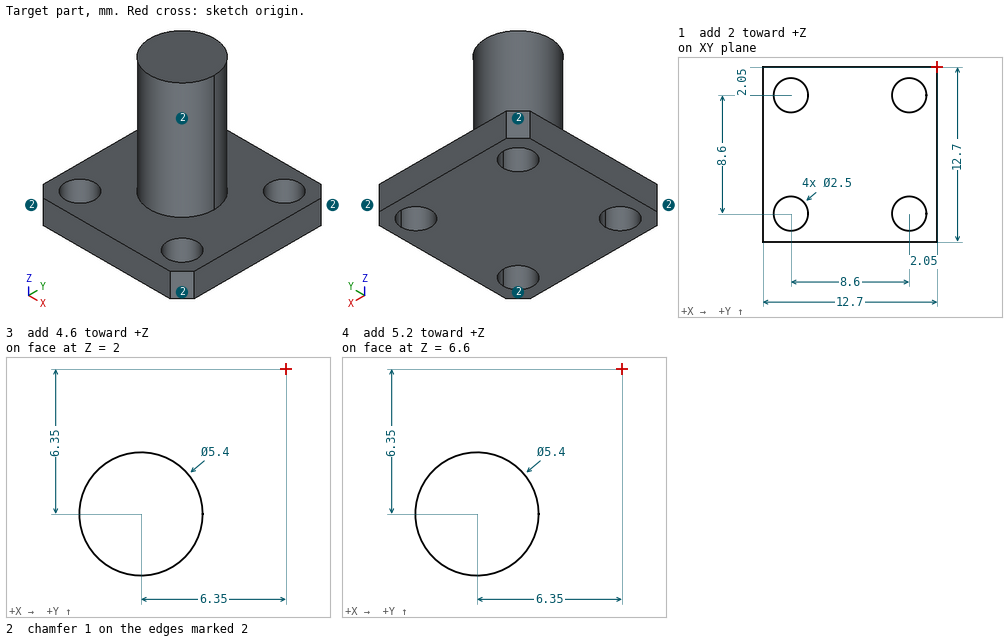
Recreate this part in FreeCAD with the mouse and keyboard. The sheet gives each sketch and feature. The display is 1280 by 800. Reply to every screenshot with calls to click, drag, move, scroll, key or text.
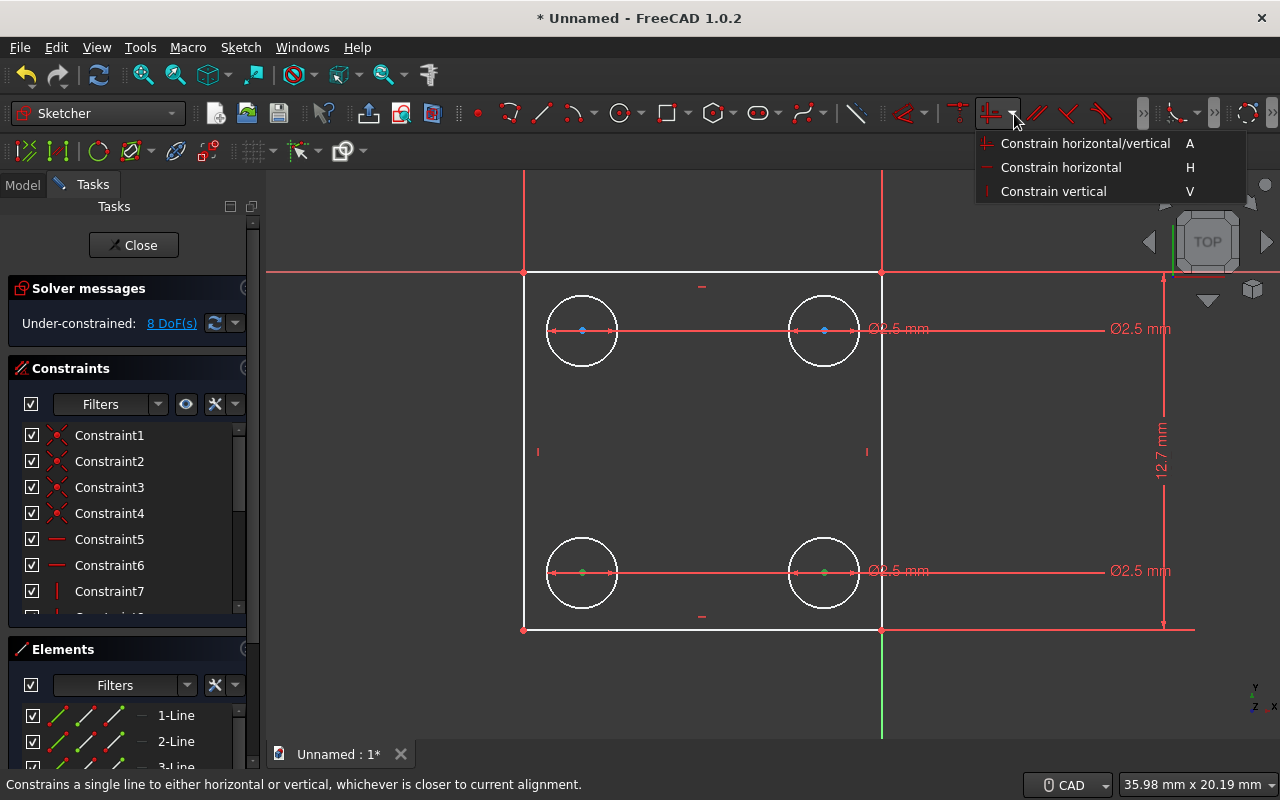
click(1111, 167)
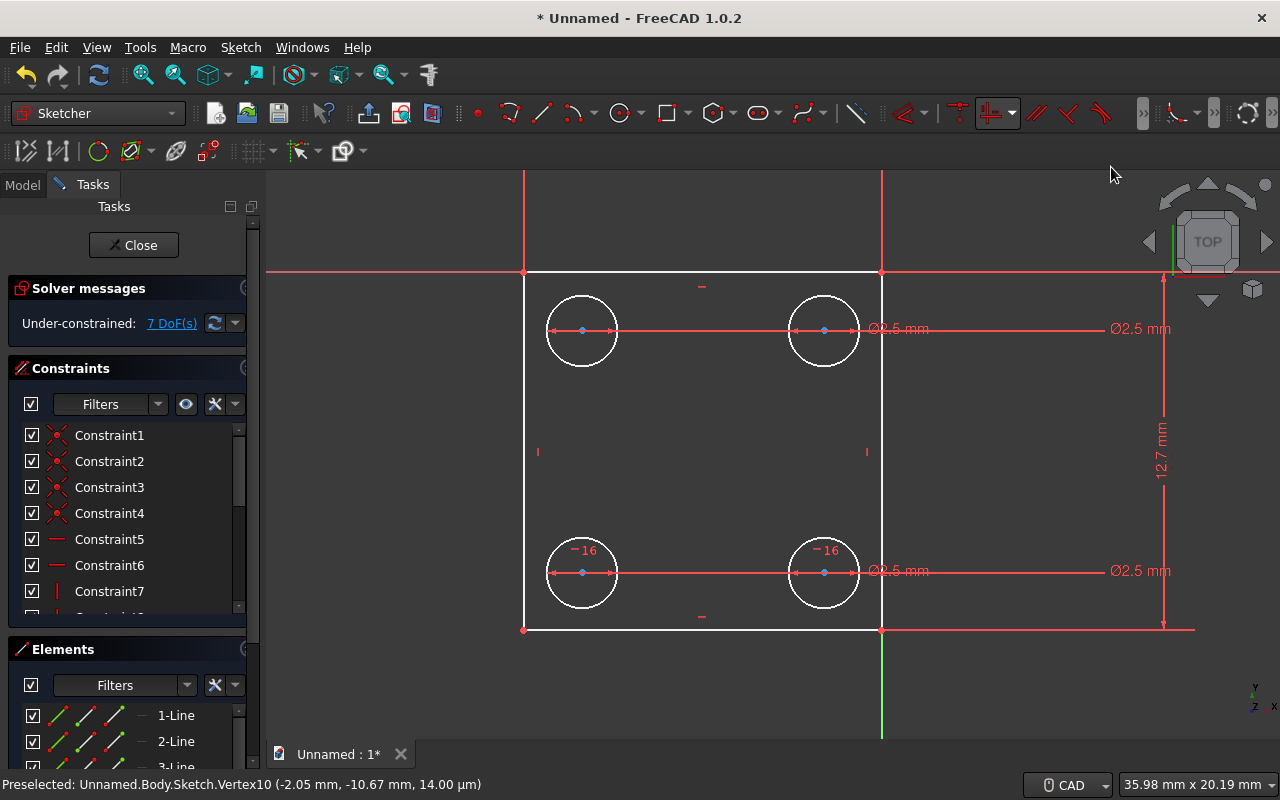
click(582, 573)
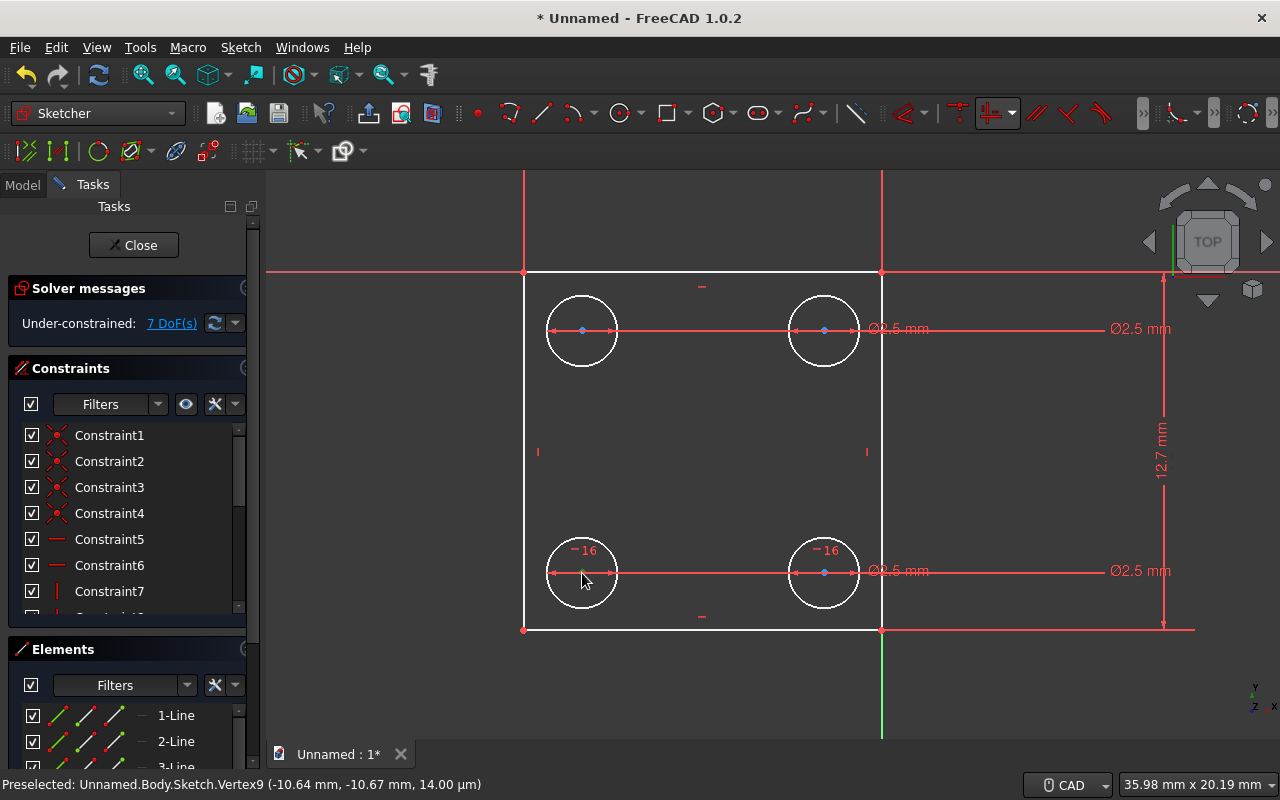
click(582, 331)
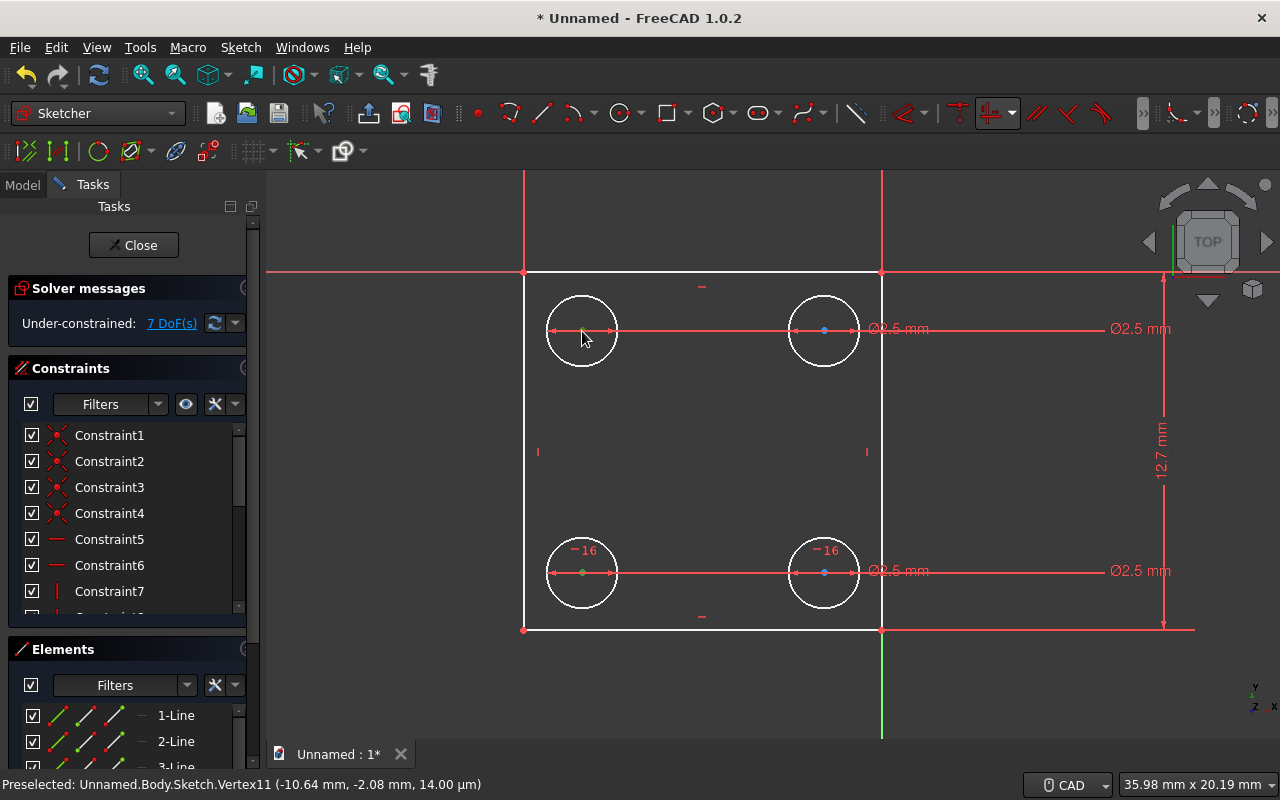
key(v)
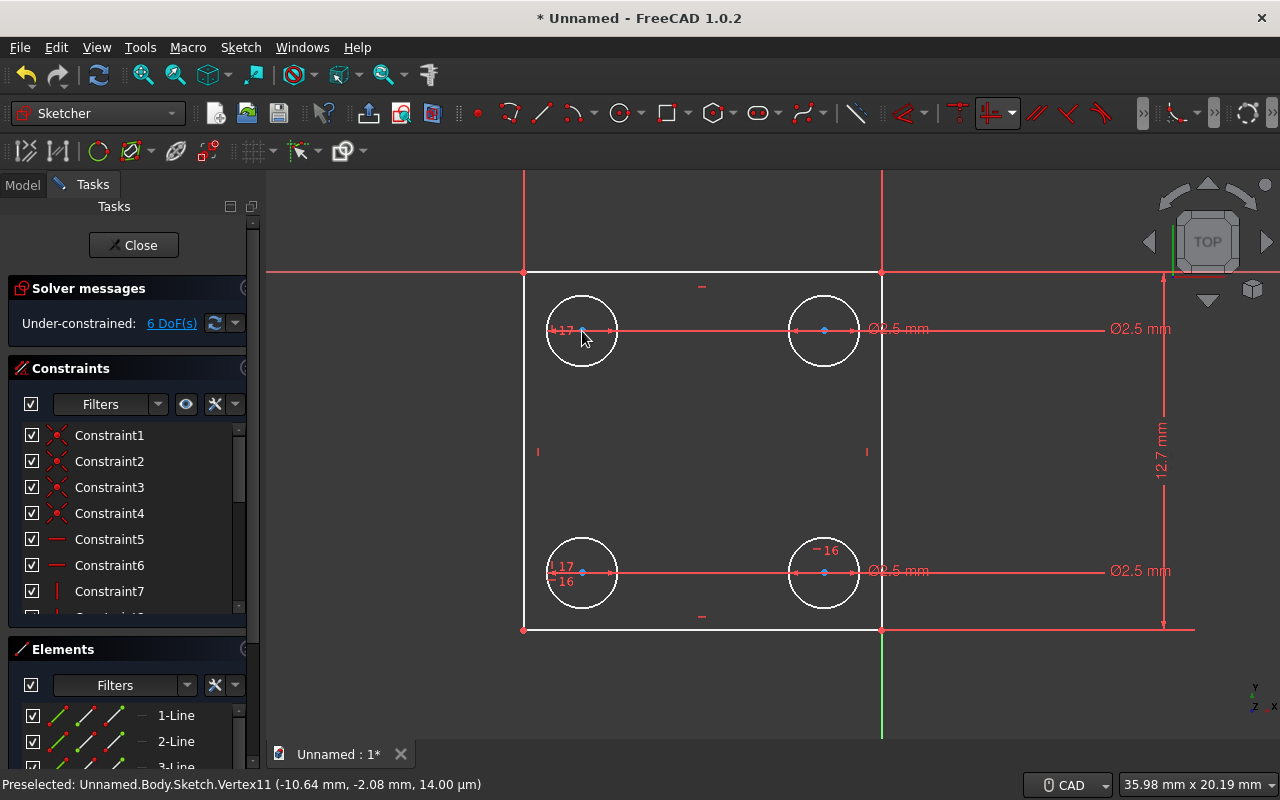
click(824, 573)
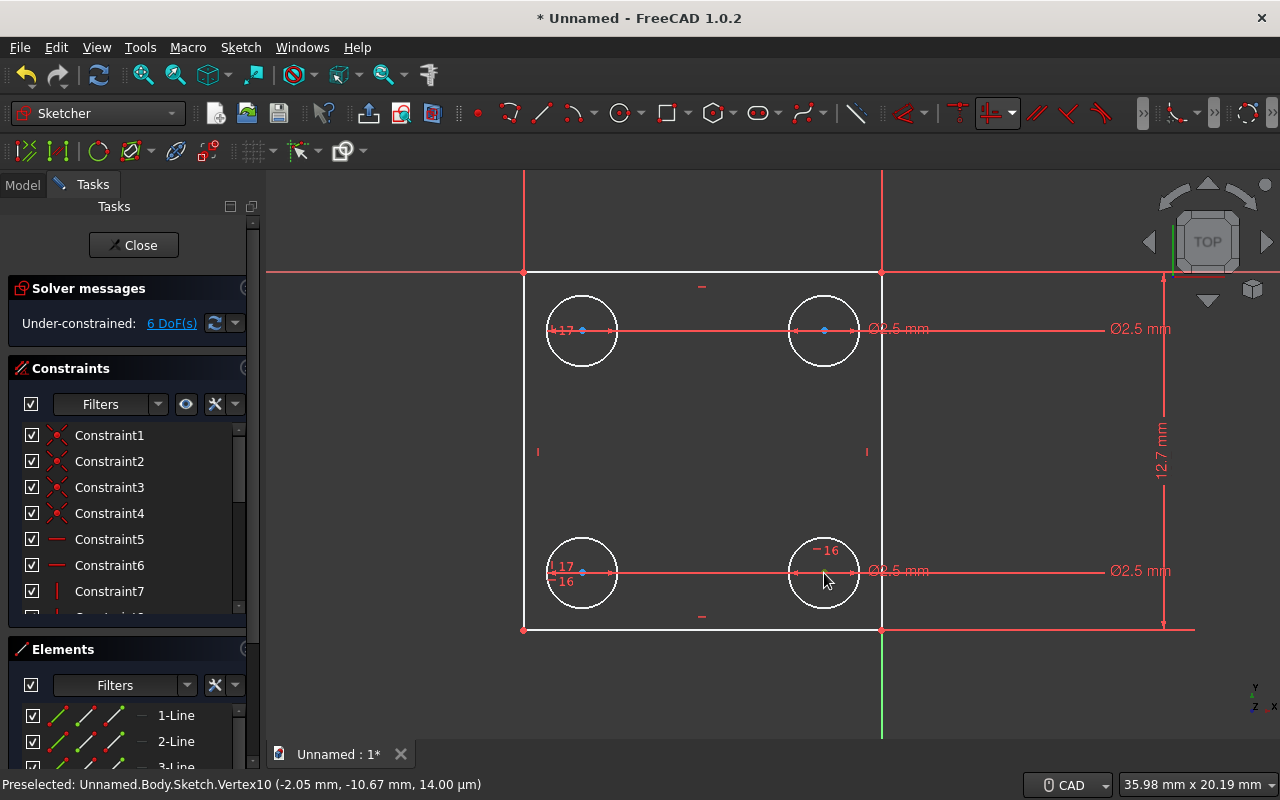
click(824, 331)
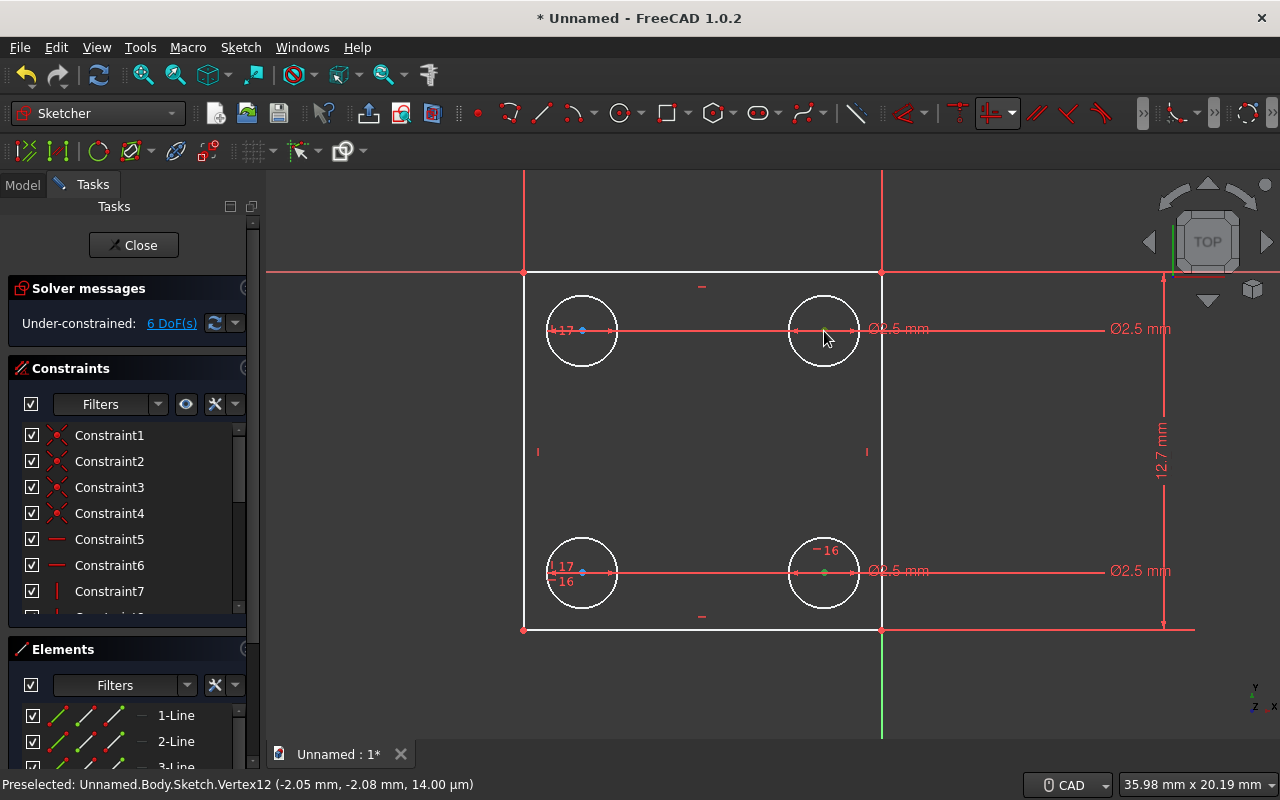
click(1014, 114)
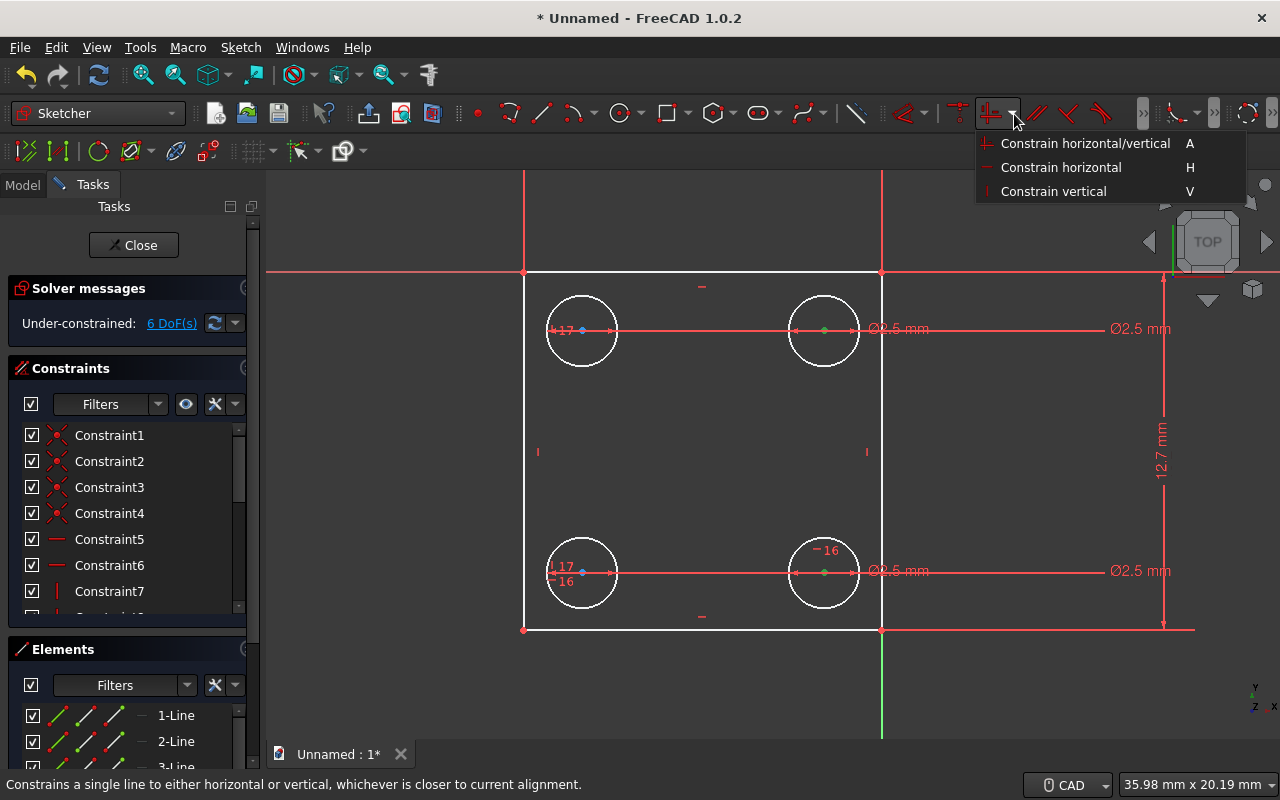
click(1111, 191)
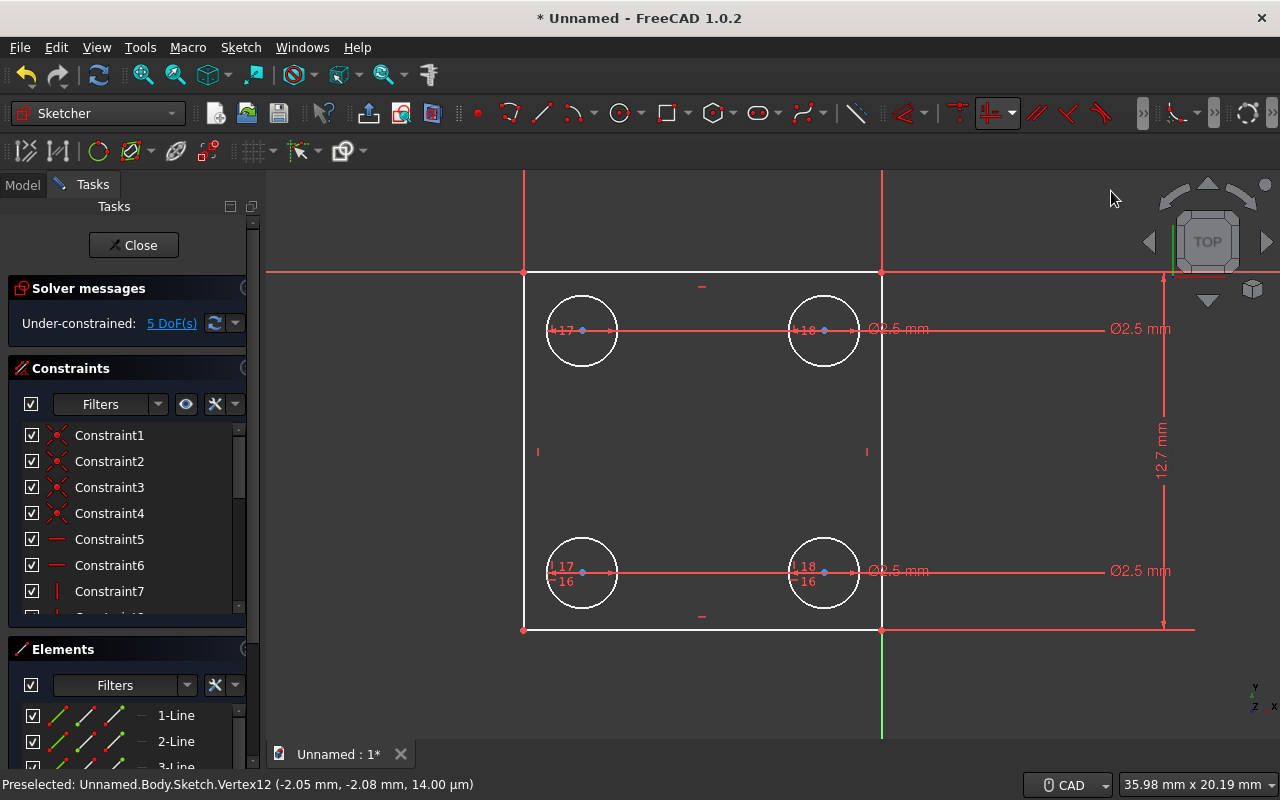
click(582, 331)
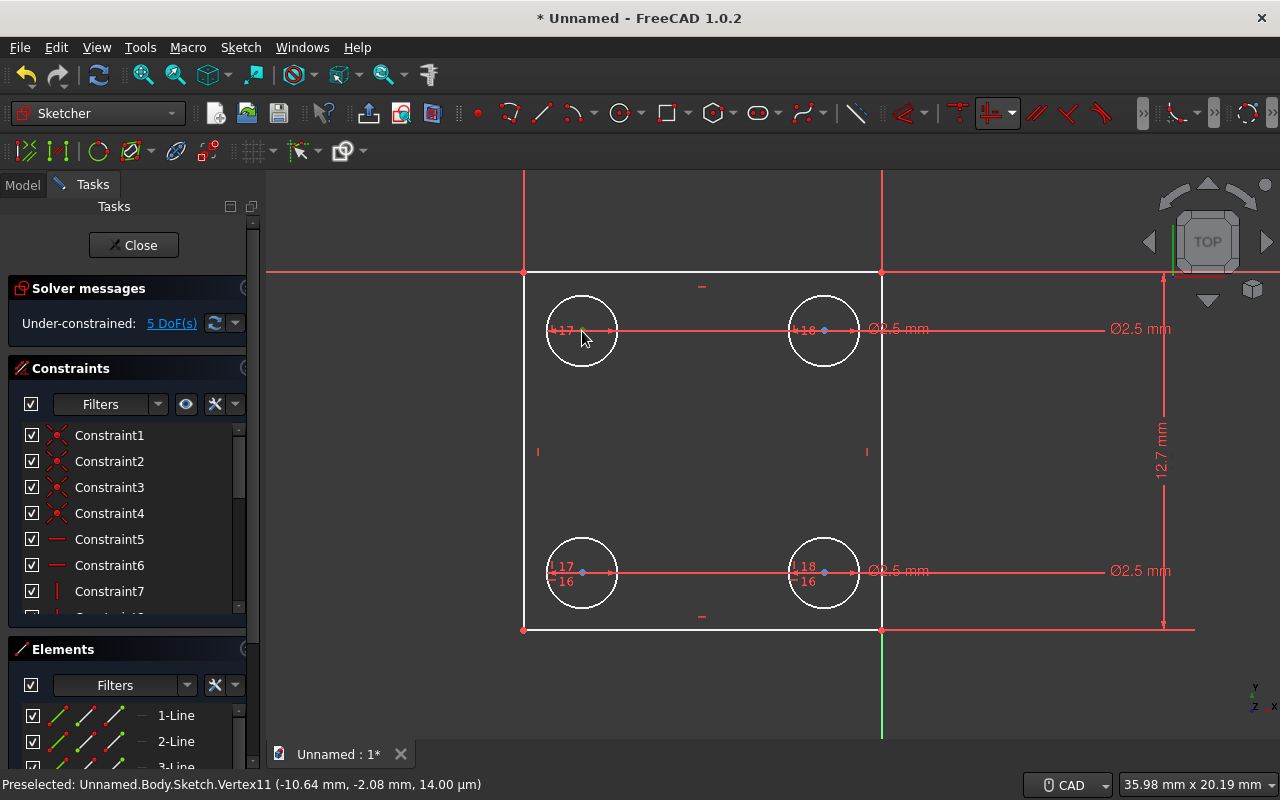
click(824, 331)